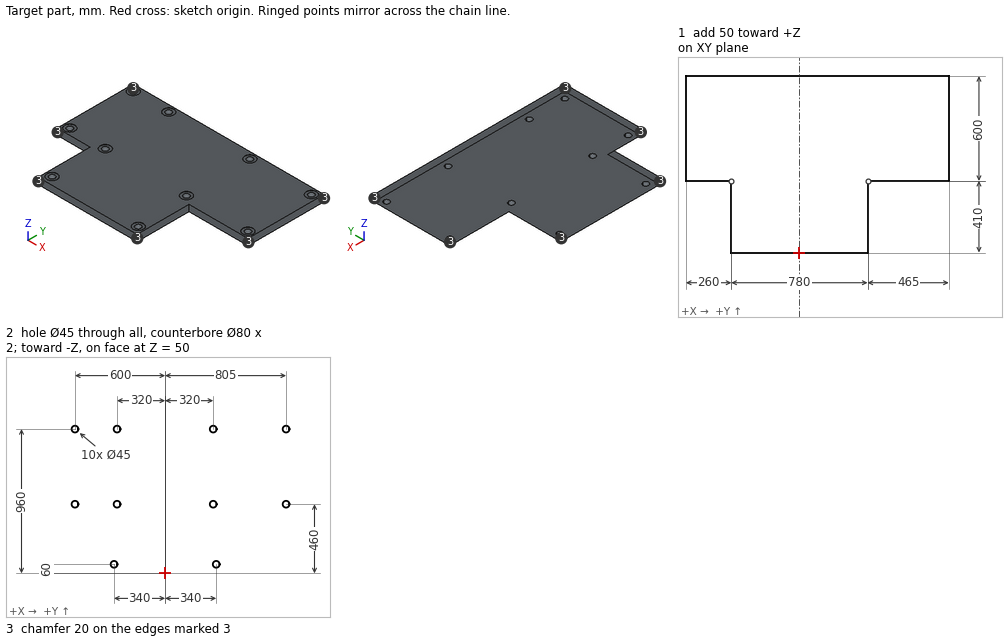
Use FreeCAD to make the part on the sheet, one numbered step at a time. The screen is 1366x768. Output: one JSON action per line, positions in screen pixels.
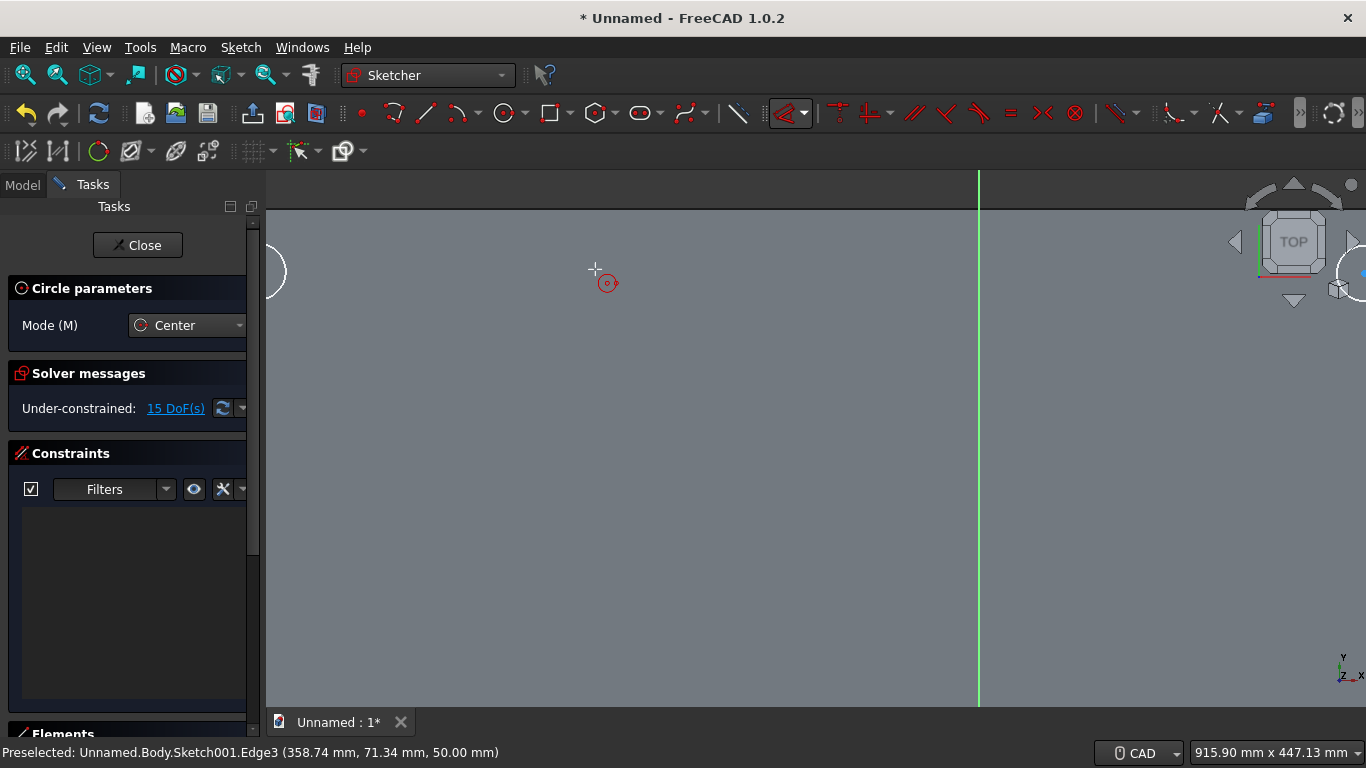
{"action": "scroll", "coordinate": [595, 269], "scroll_direction": "down", "scroll_amount": 6}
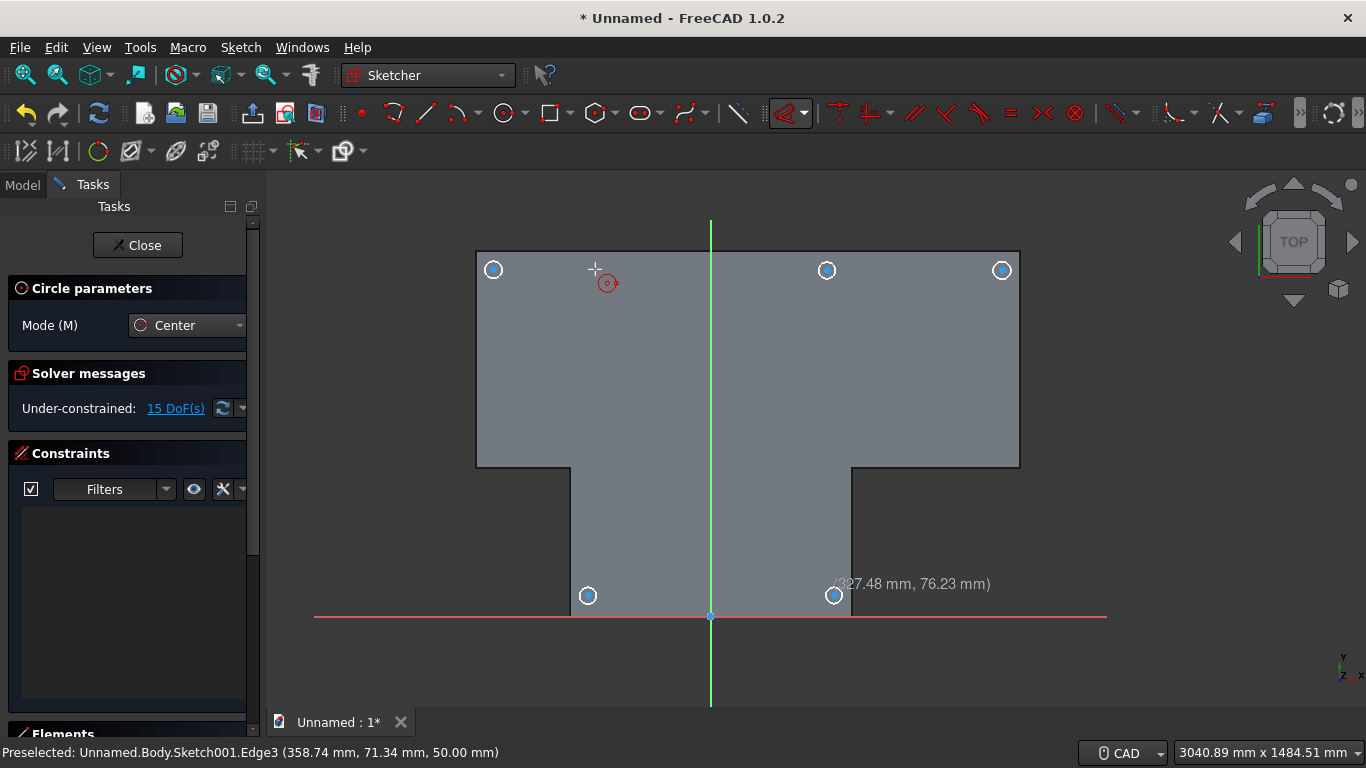
{"action": "left_click", "coordinate": [595, 269]}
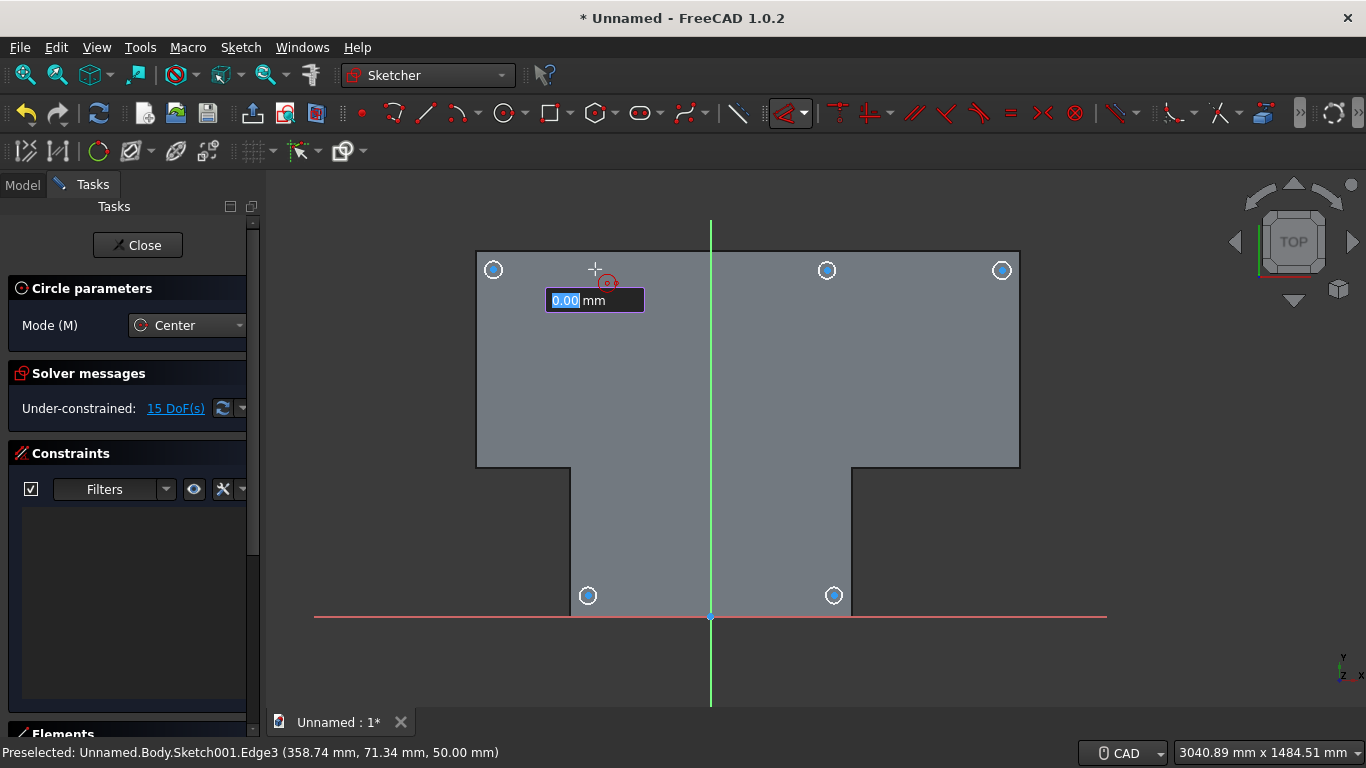
{"action": "scroll", "coordinate": [601, 263], "scroll_direction": "up", "scroll_amount": 4}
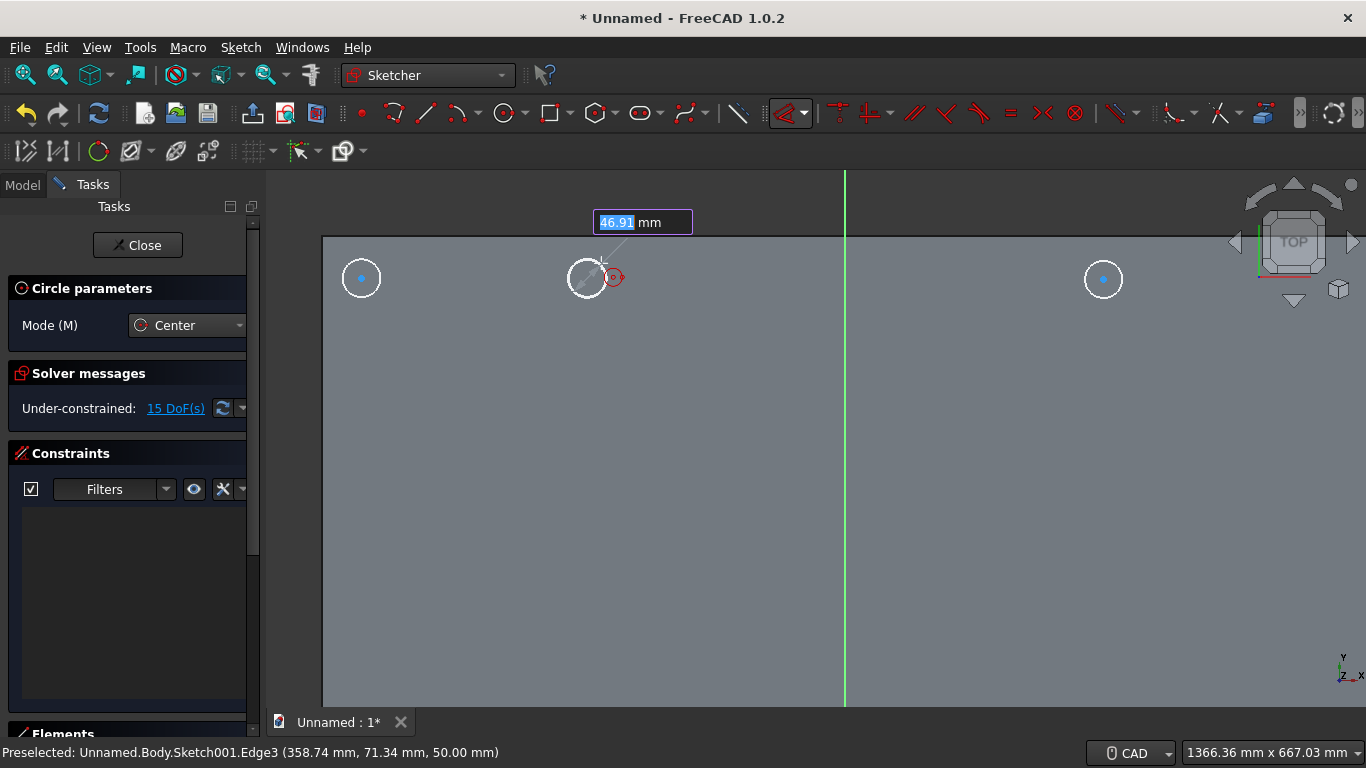
{"action": "left_click", "coordinate": [600, 264]}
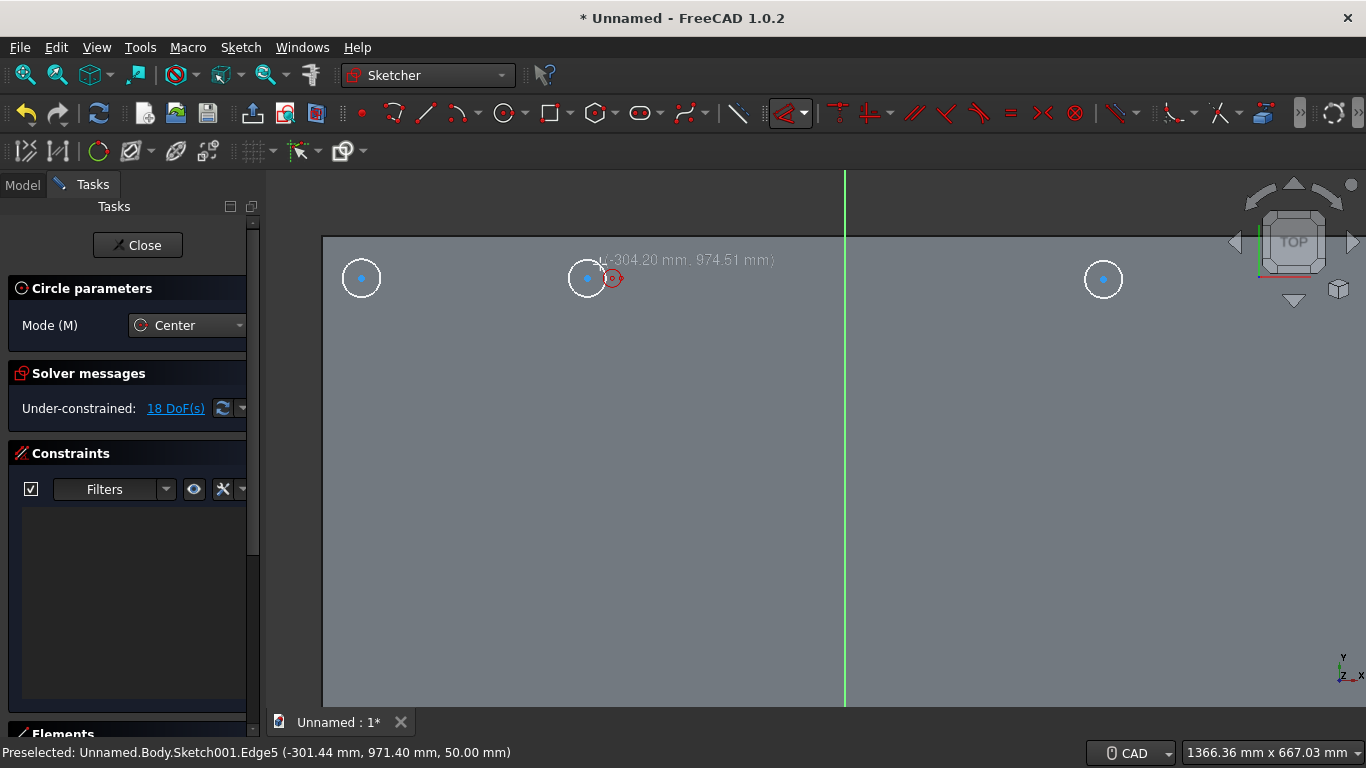
{"action": "scroll", "coordinate": [601, 263], "scroll_direction": "down", "scroll_amount": 4}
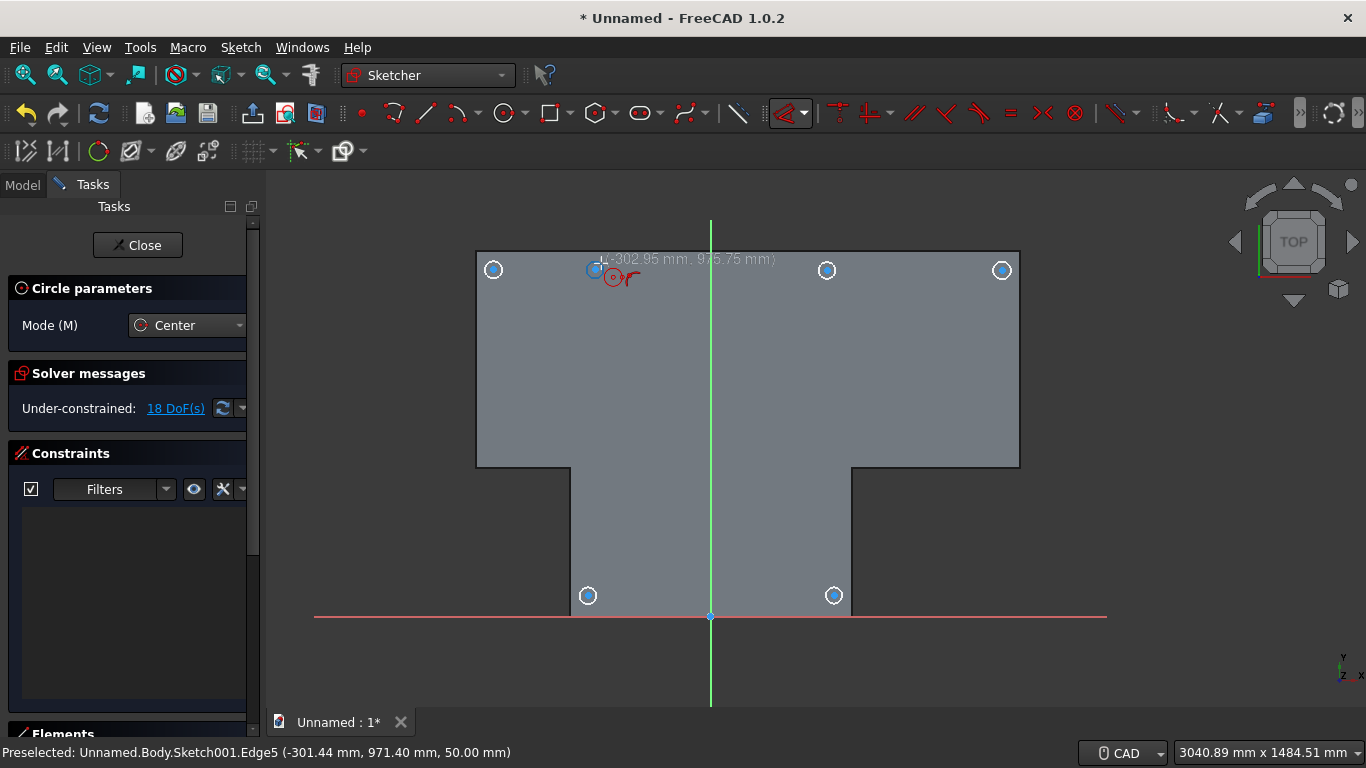
{"action": "scroll", "coordinate": [1002, 450], "scroll_direction": "up", "scroll_amount": 6}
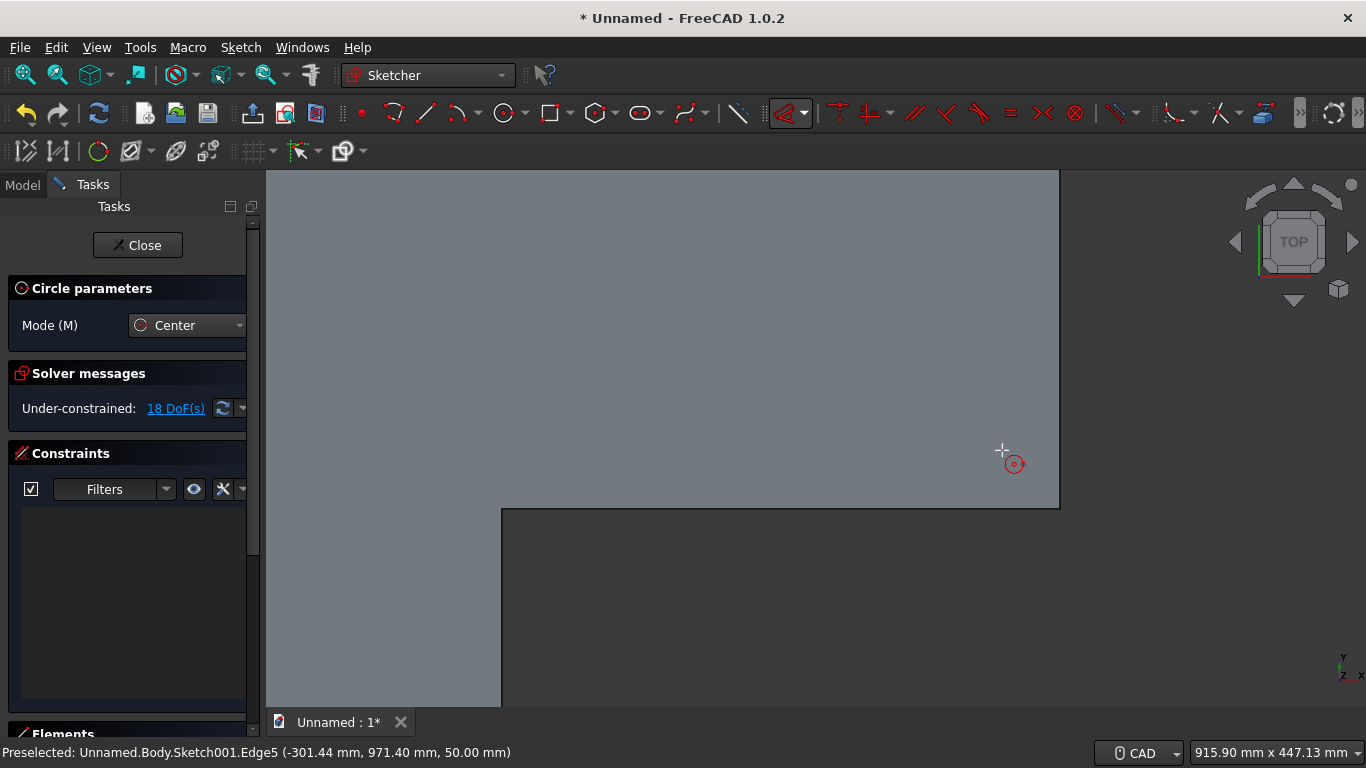
{"action": "scroll", "coordinate": [1002, 450], "scroll_direction": "down", "scroll_amount": 6}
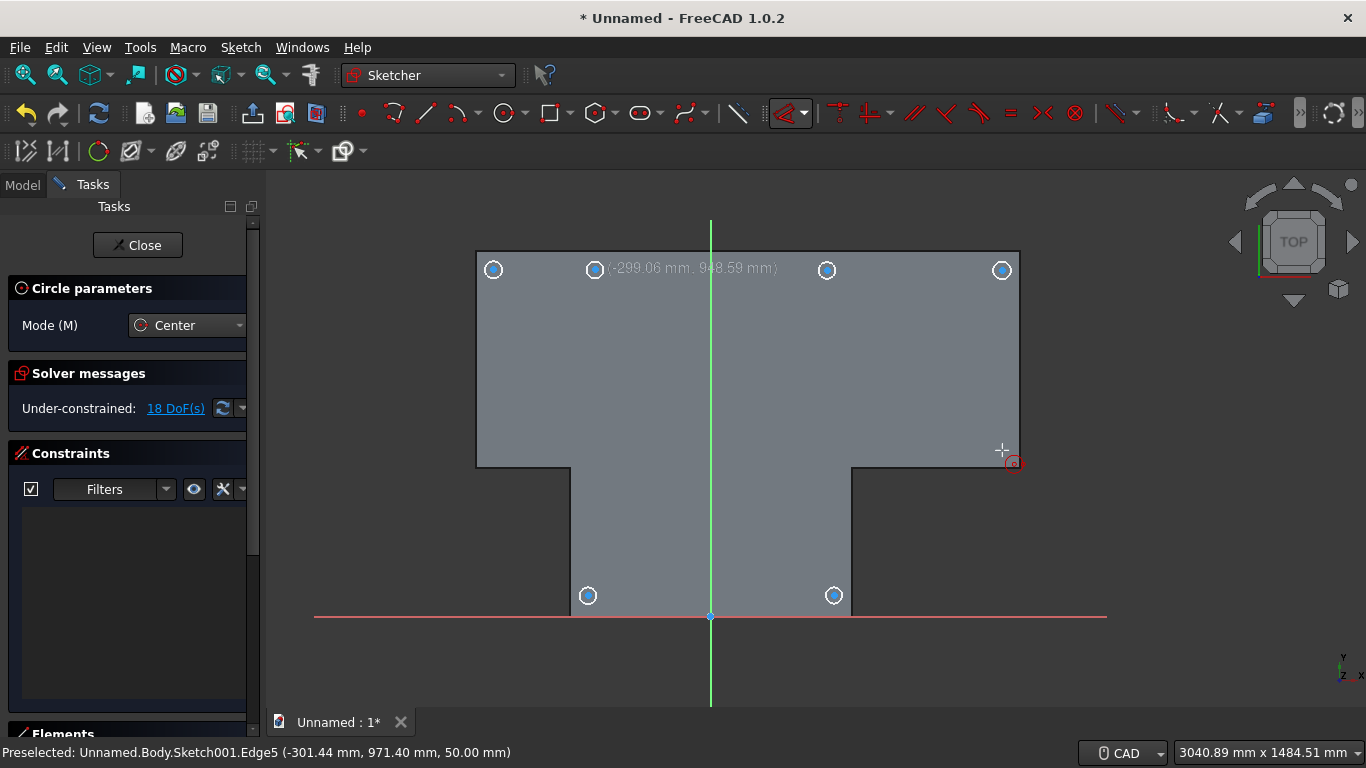
{"action": "left_click", "coordinate": [1002, 450]}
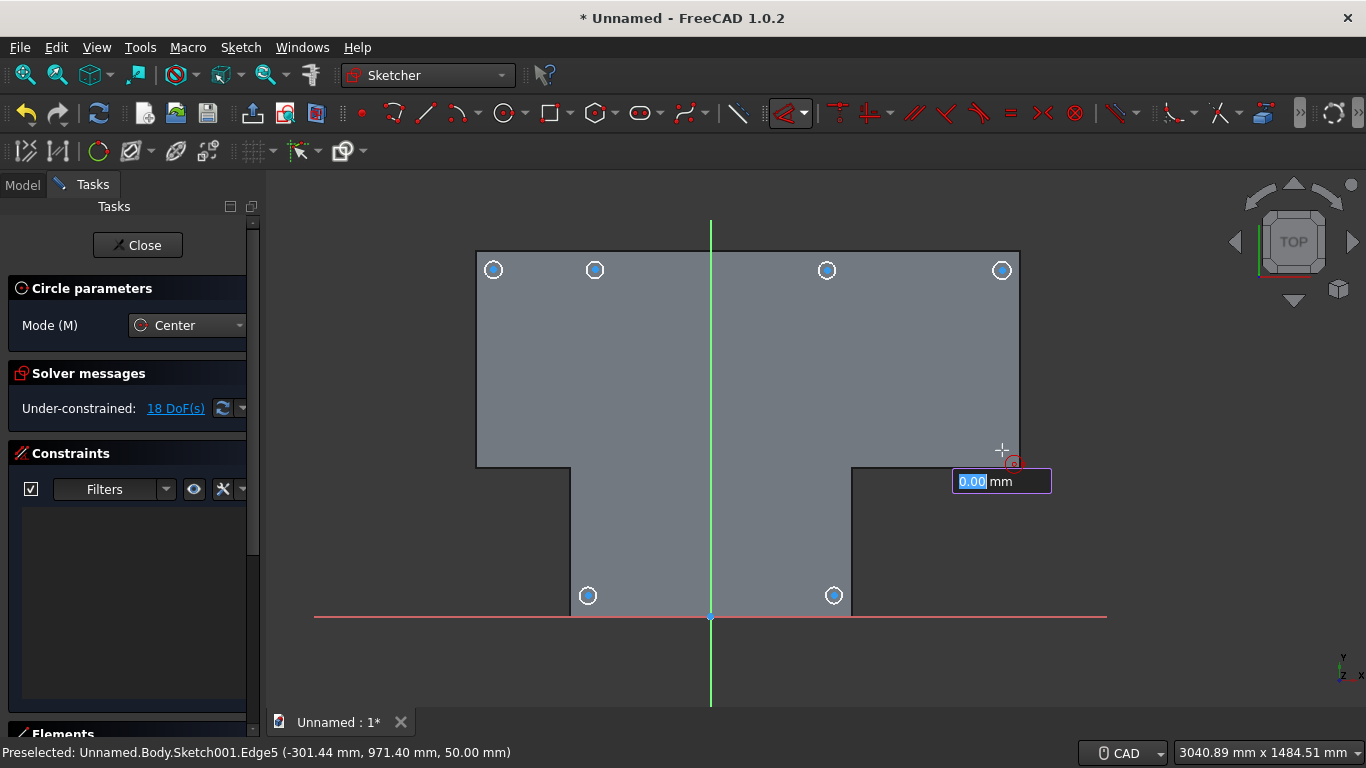
{"action": "scroll", "coordinate": [1008, 444], "scroll_direction": "up", "scroll_amount": 4}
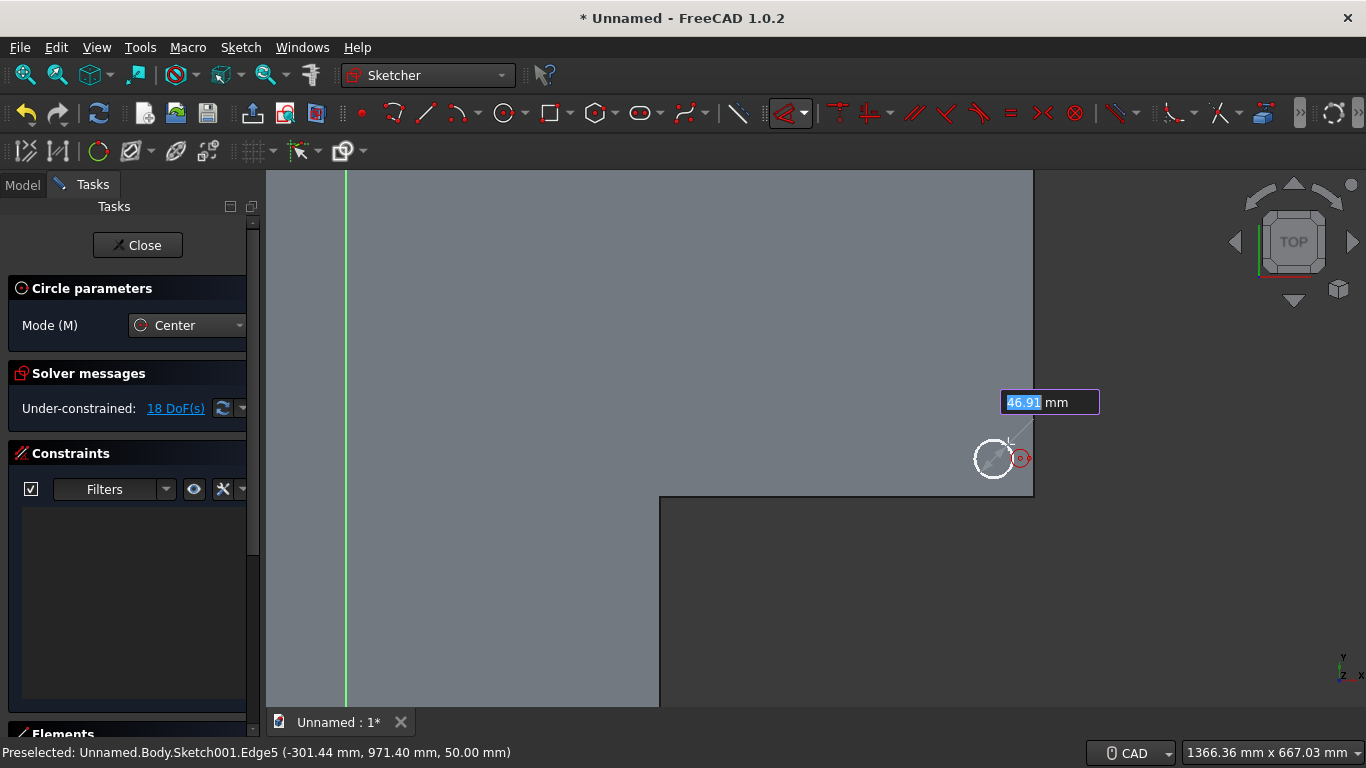
{"action": "left_click", "coordinate": [1007, 444]}